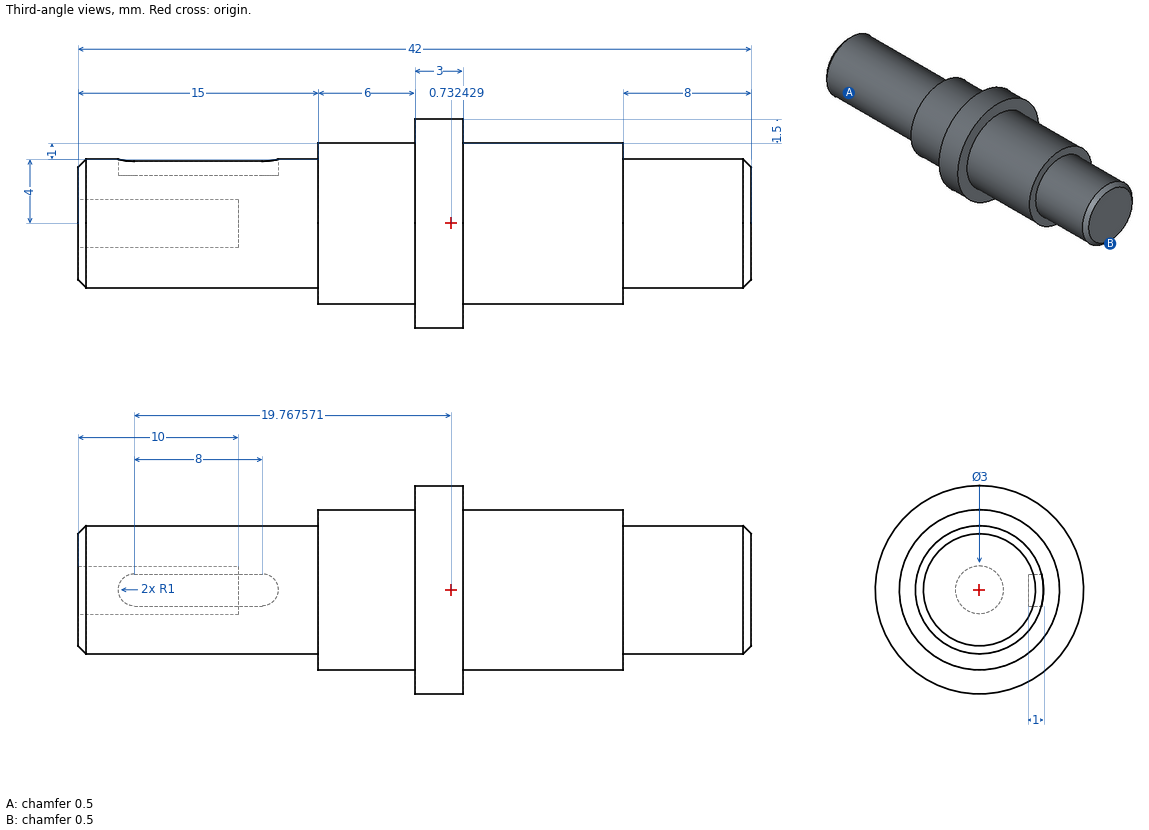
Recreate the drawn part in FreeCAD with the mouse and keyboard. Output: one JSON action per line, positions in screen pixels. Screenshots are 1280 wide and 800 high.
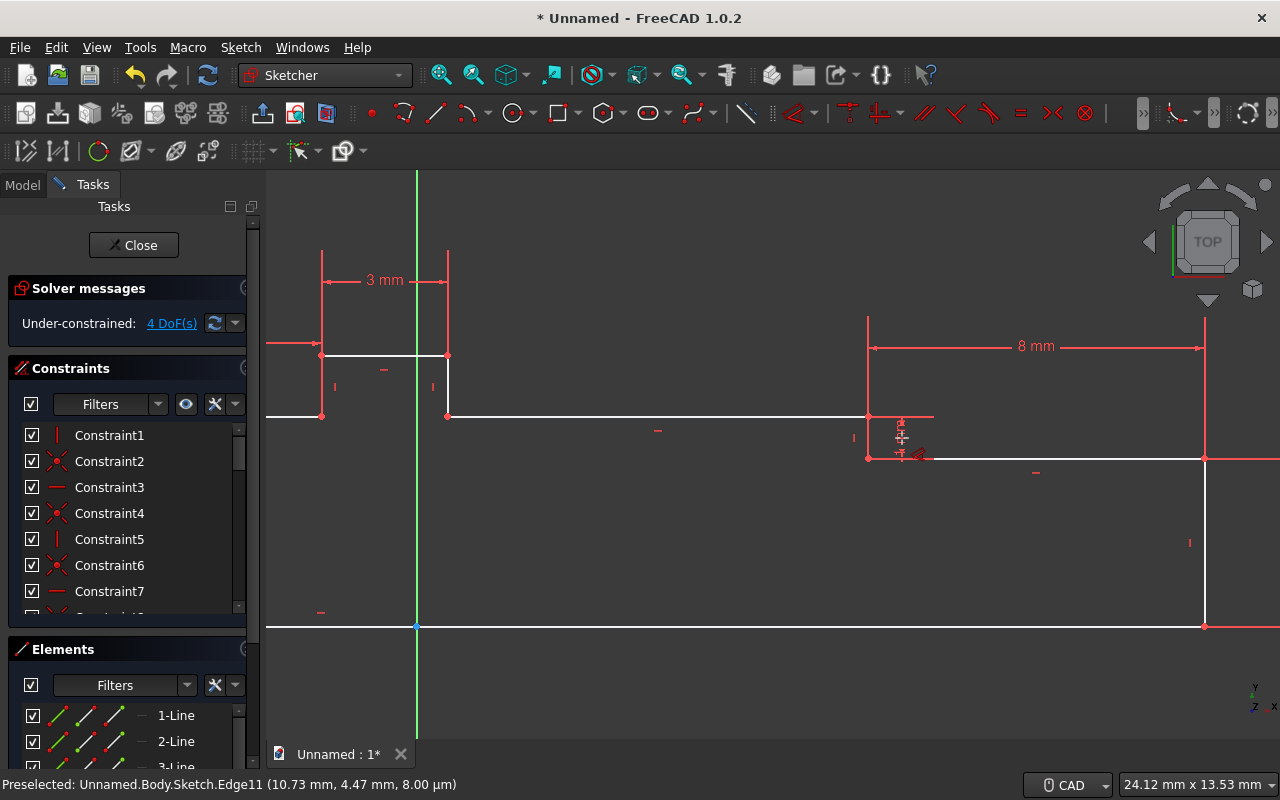
{"action": "scroll", "coordinate": [870, 439], "scroll_direction": "down", "scroll_amount": 6}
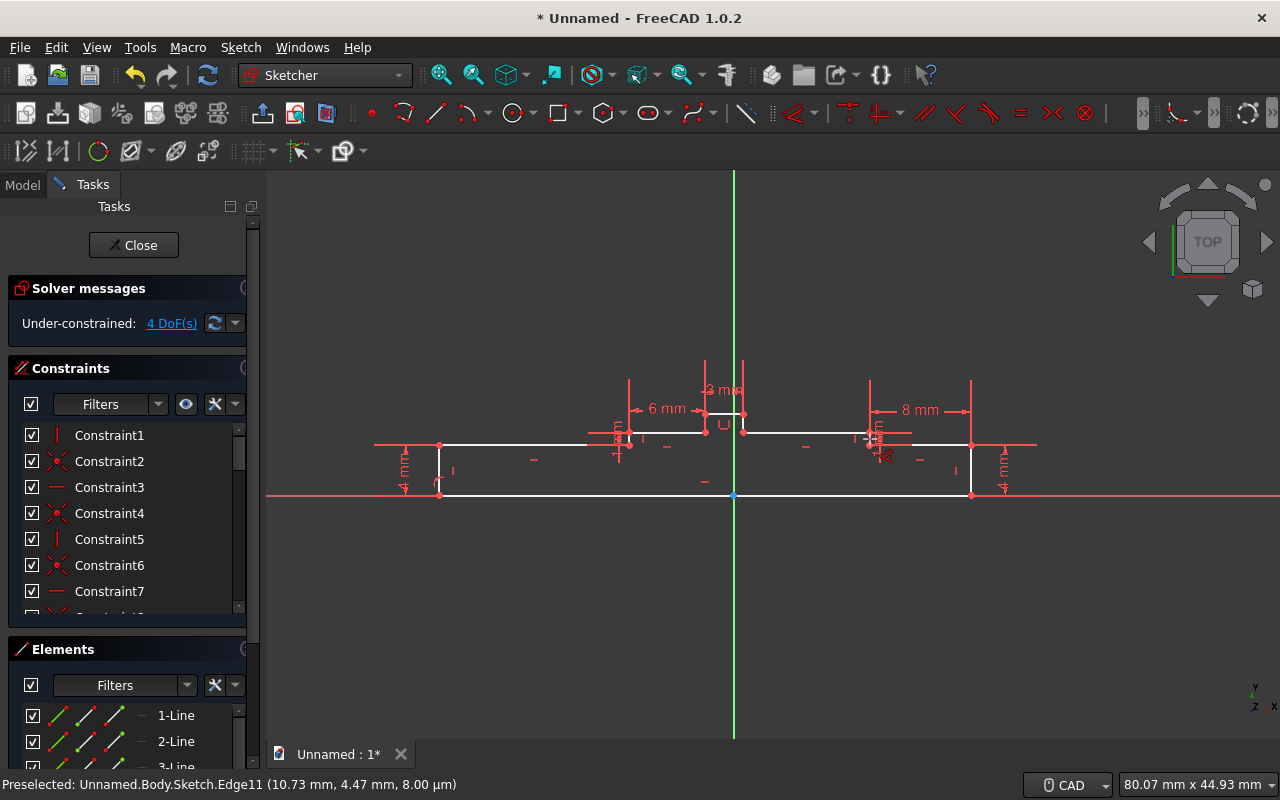
{"action": "left_click", "coordinate": [572, 445]}
{"action": "left_click", "coordinate": [534, 411]}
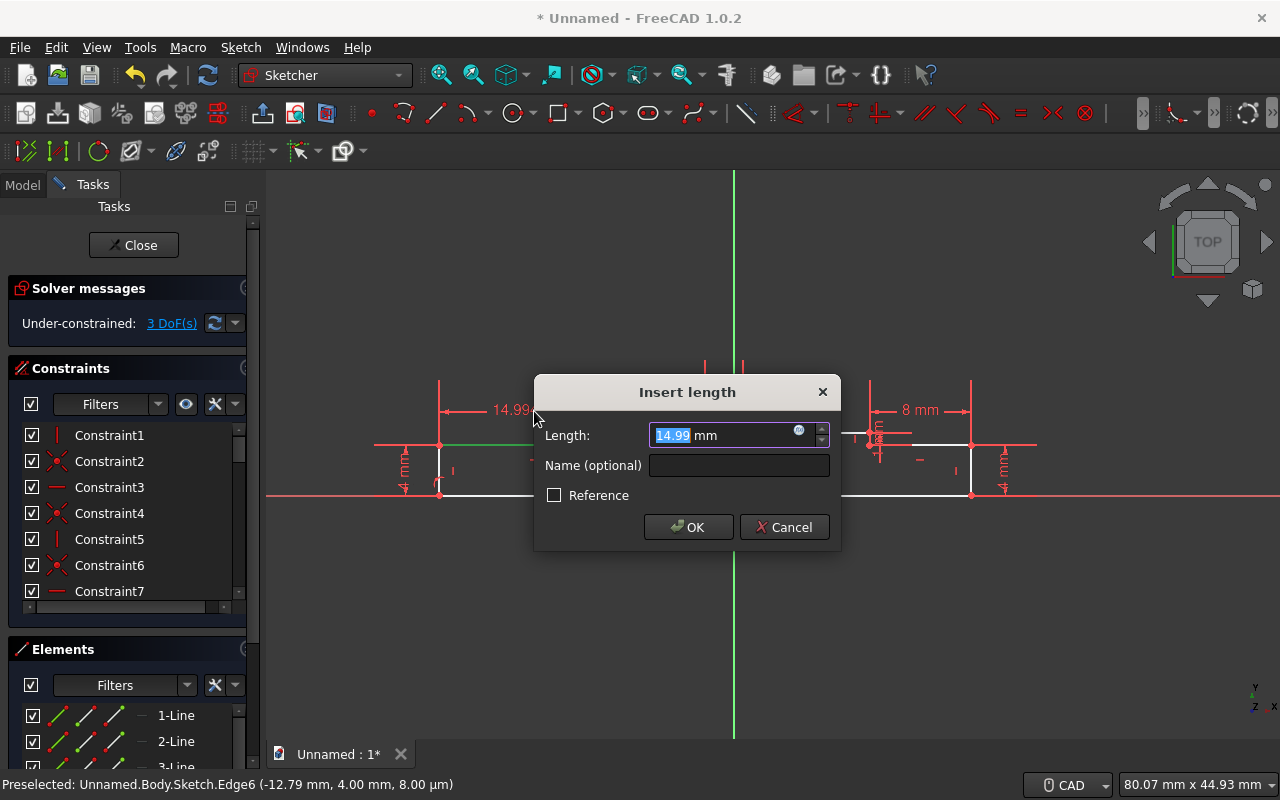
{"action": "type", "text": "15"}
{"action": "key", "text": "Return"}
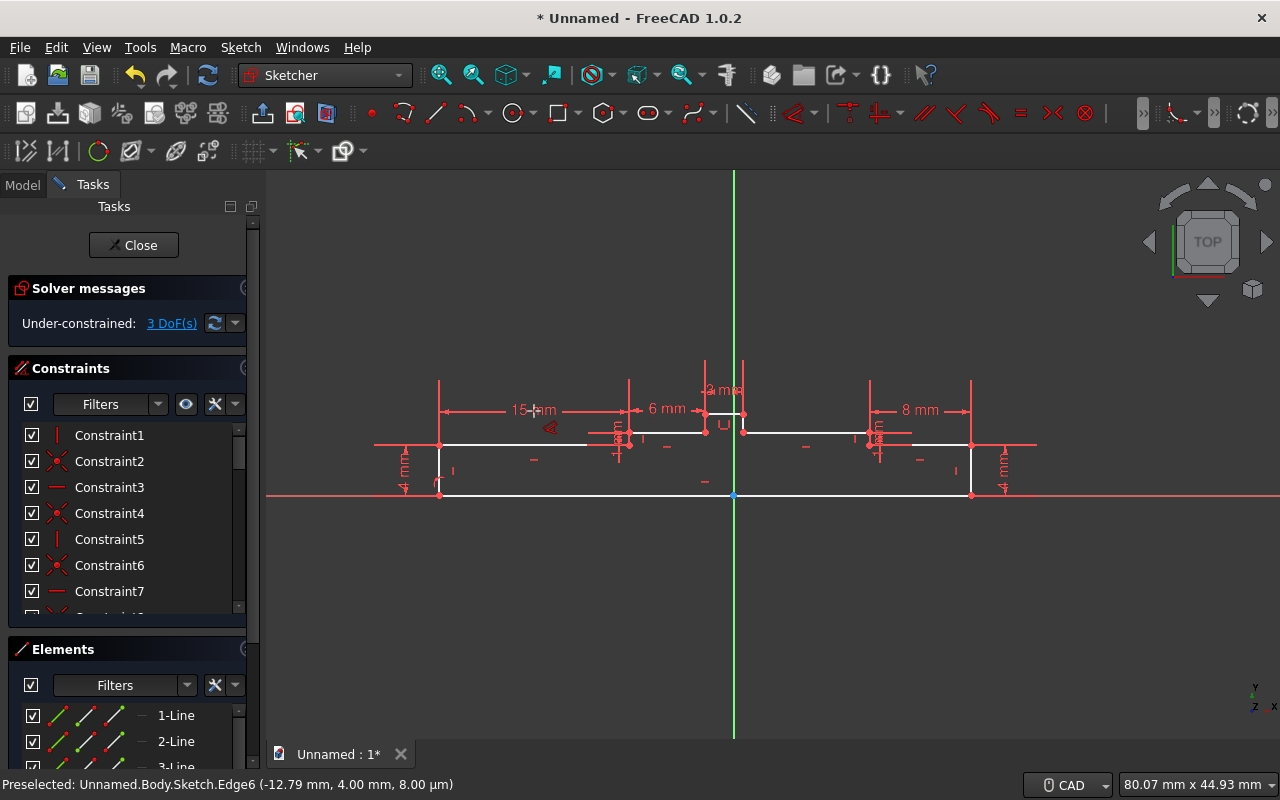
{"action": "left_click", "coordinate": [599, 496]}
{"action": "left_click", "coordinate": [705, 530]}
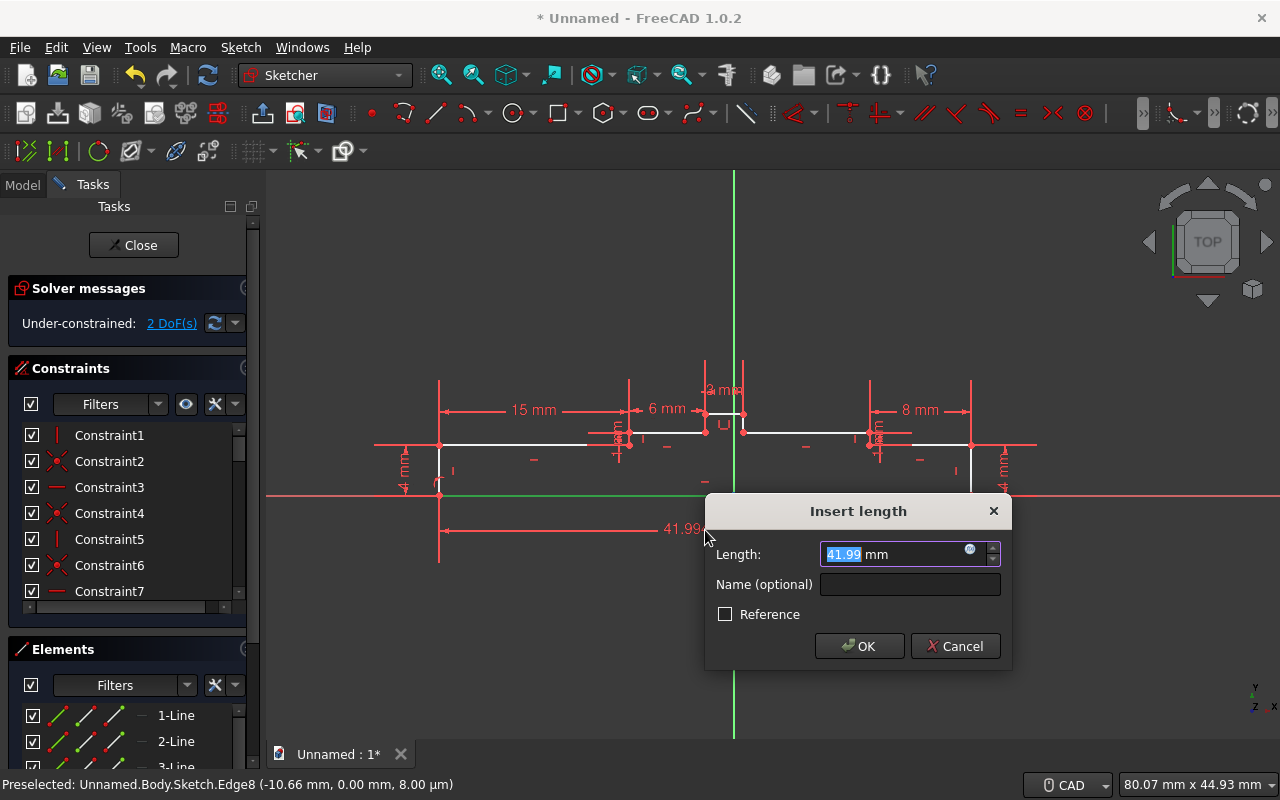
{"action": "type", "text": "42"}
{"action": "key", "text": "Return"}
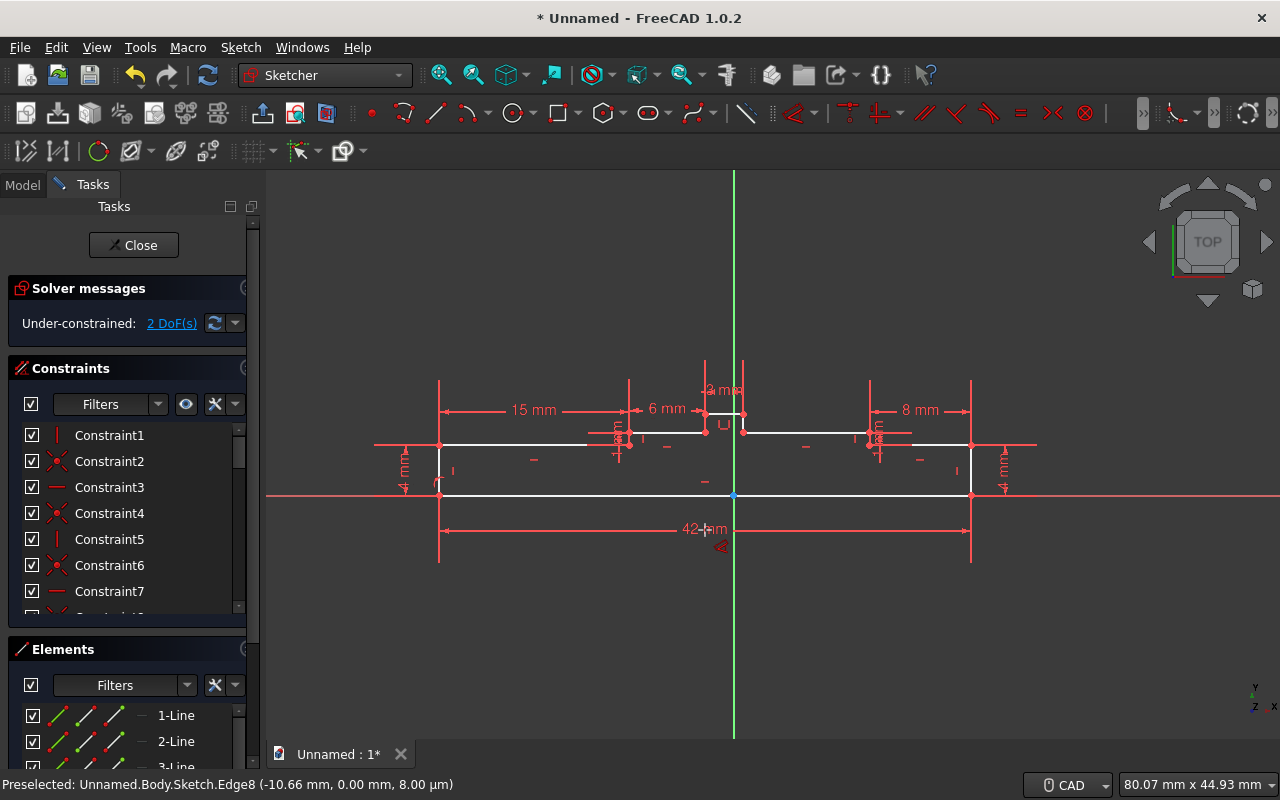
{"action": "scroll", "coordinate": [743, 423], "scroll_direction": "up", "scroll_amount": 4}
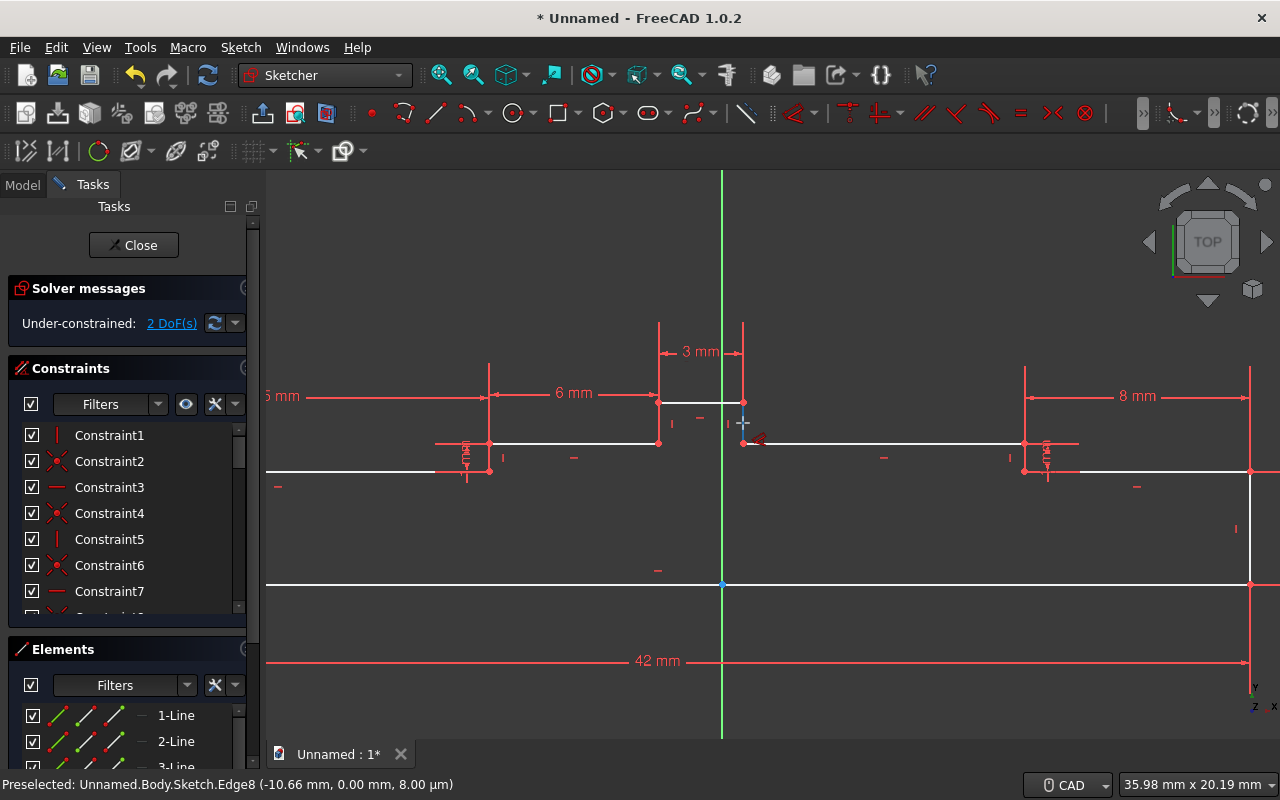
{"action": "left_click", "coordinate": [743, 423]}
{"action": "left_click", "coordinate": [777, 423]}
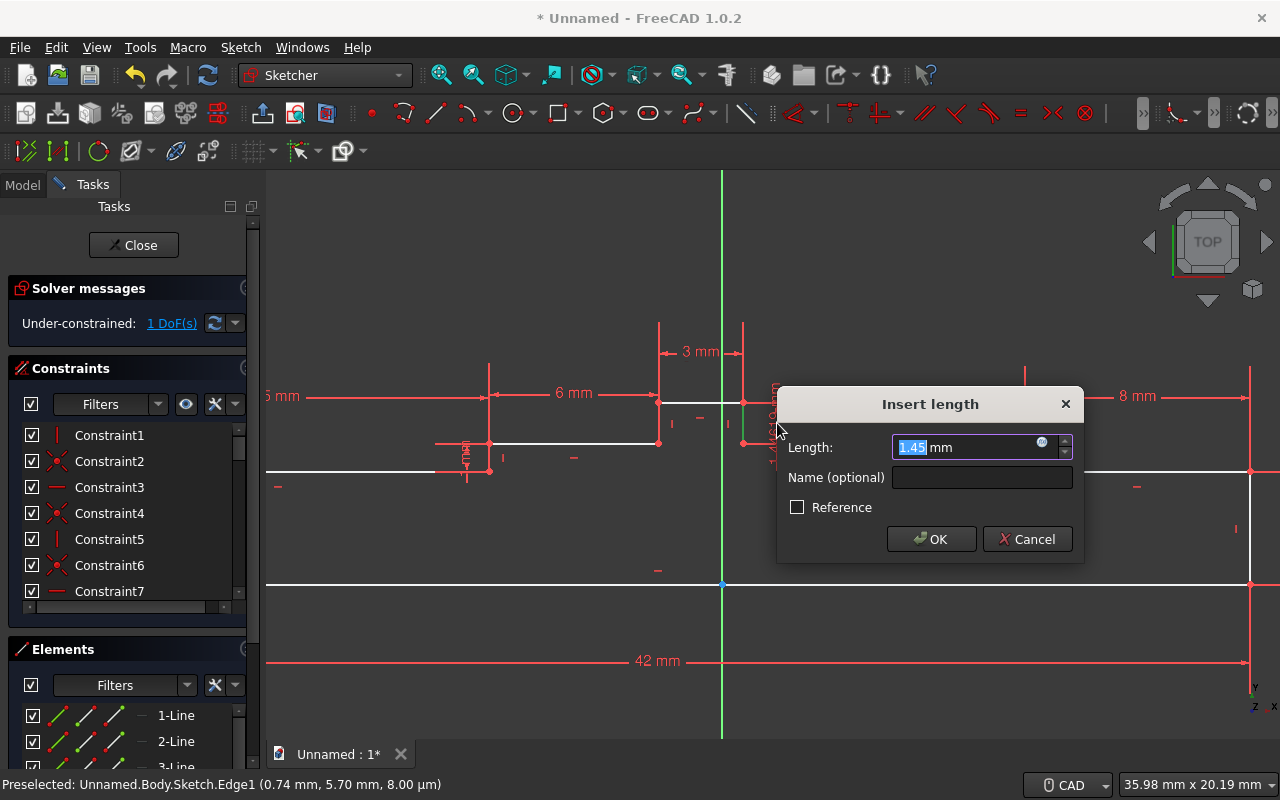
{"action": "type", "text": "1.5"}
{"action": "key", "text": "Return"}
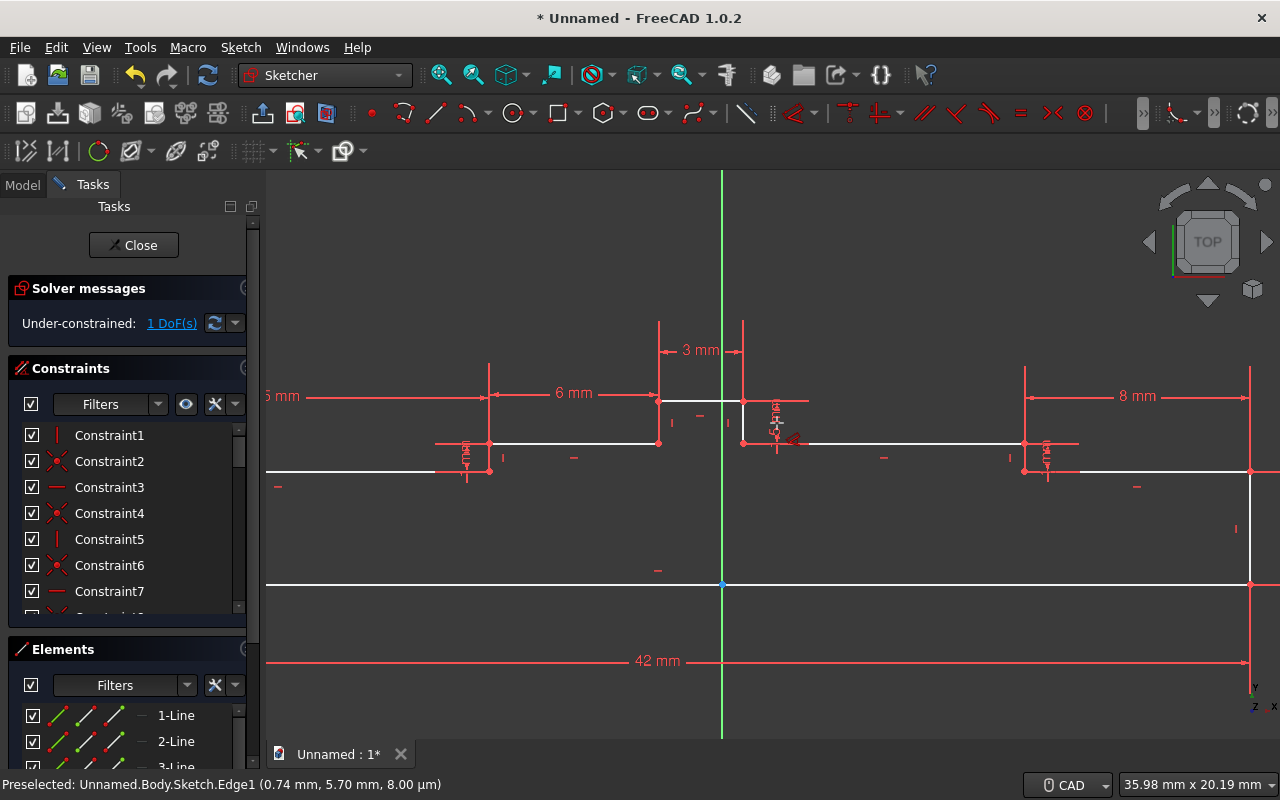
{"action": "scroll", "coordinate": [743, 444], "scroll_direction": "up", "scroll_amount": 4}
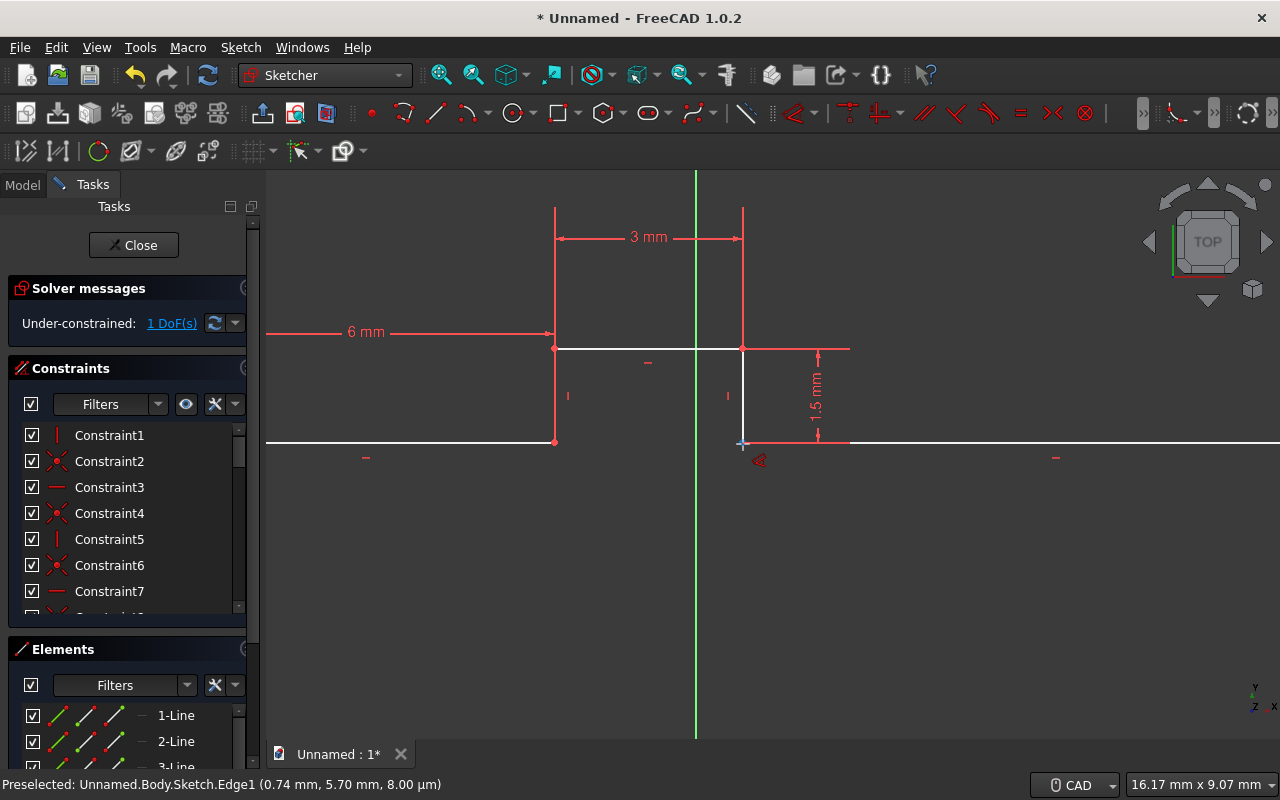
{"action": "left_click", "coordinate": [743, 443]}
{"action": "left_click", "coordinate": [720, 409]}